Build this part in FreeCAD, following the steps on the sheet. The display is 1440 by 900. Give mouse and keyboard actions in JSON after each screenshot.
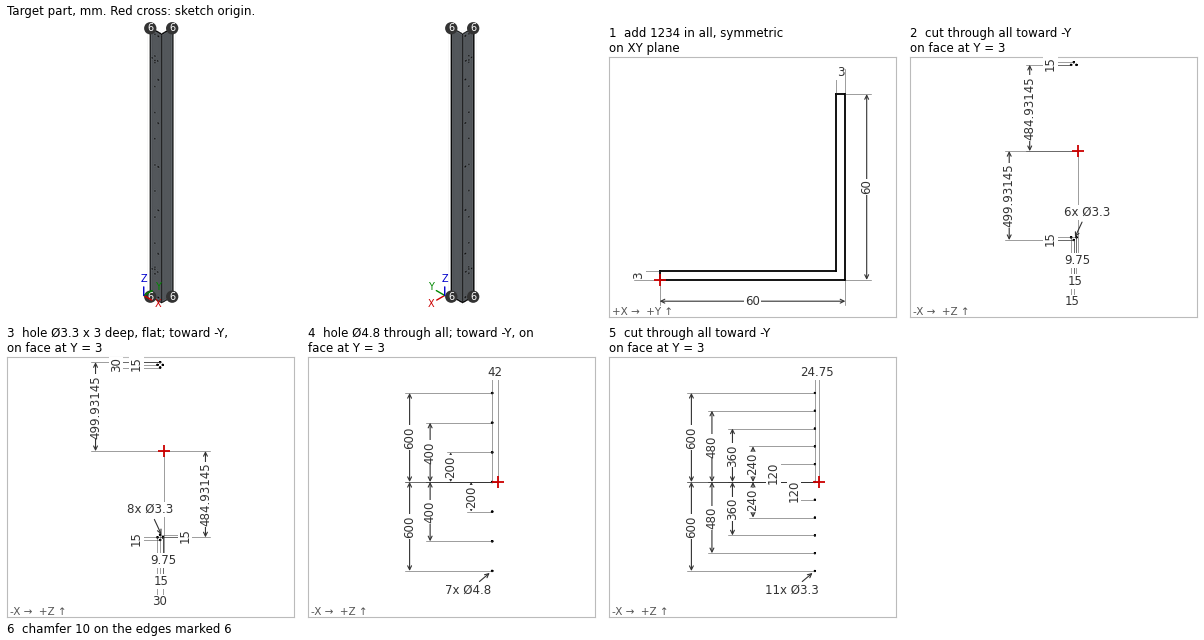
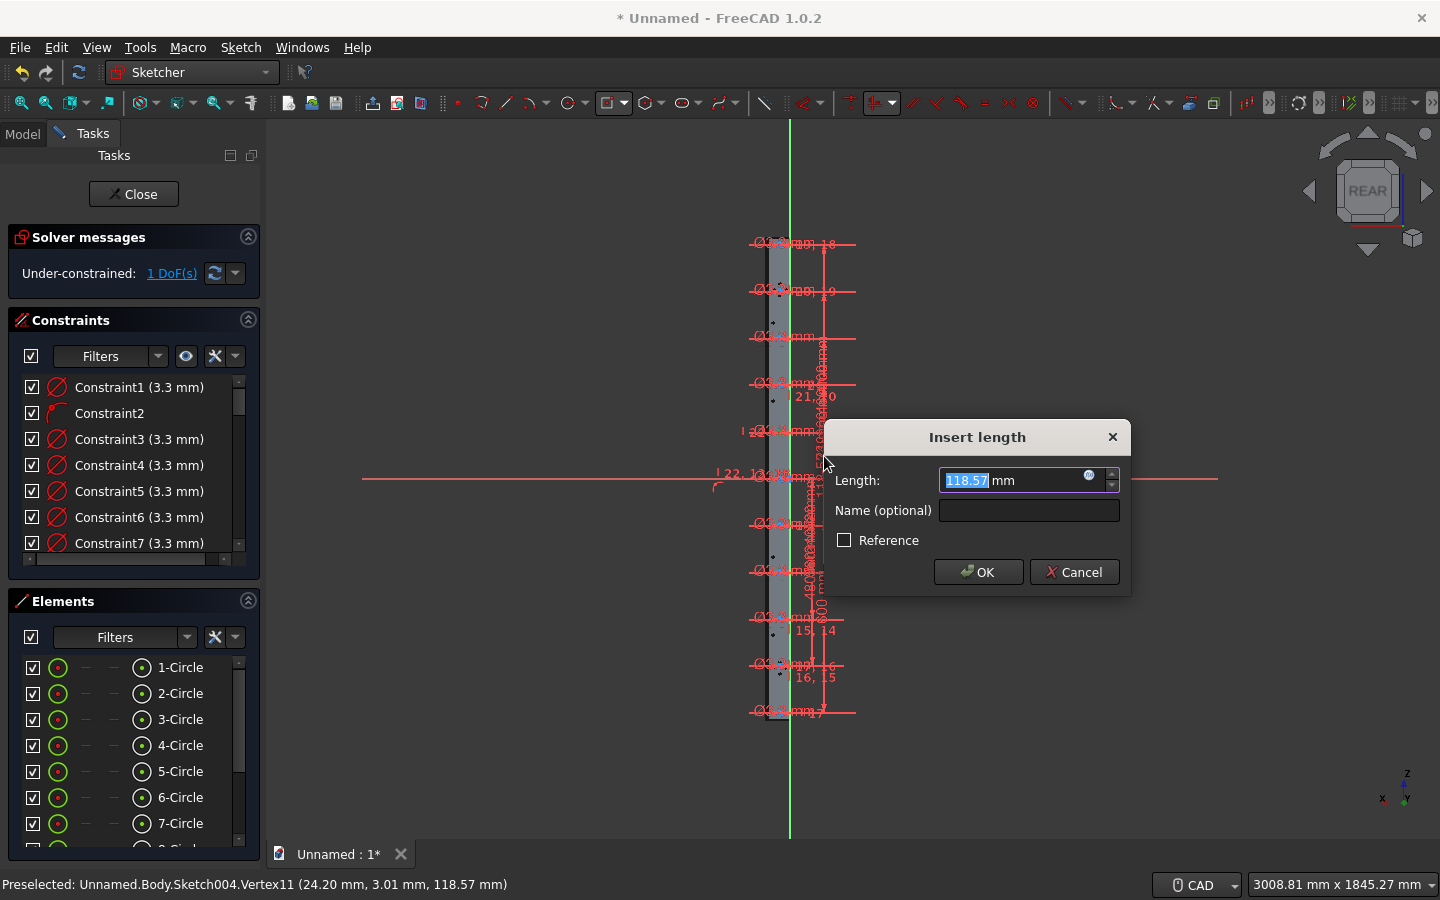
{"action": "type", "text": "120"}
{"action": "key", "text": "Return"}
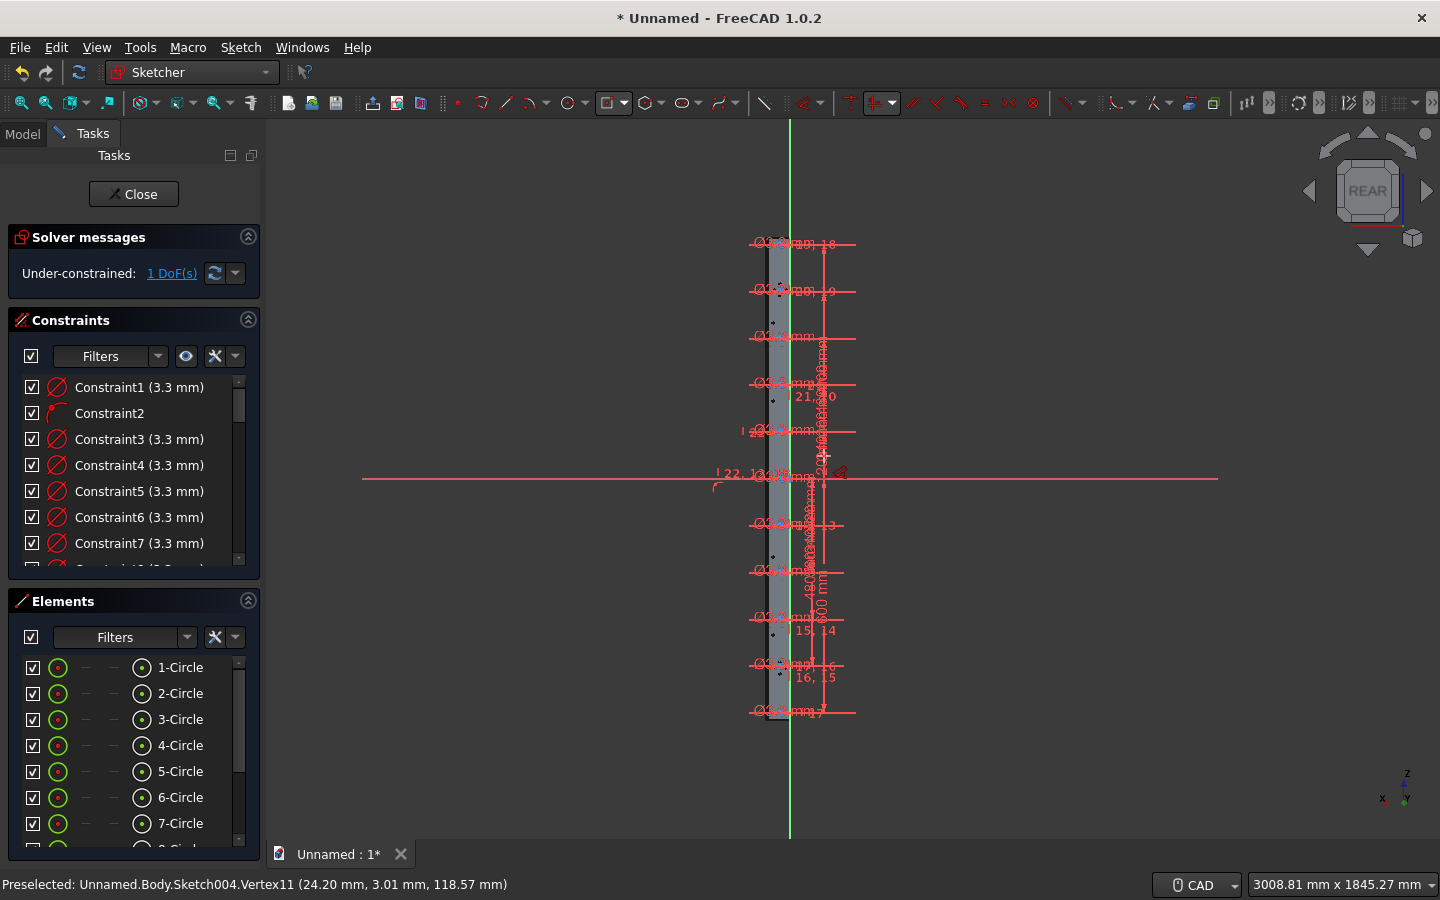
{"action": "scroll", "coordinate": [780, 479], "scroll_direction": "up", "scroll_amount": 8}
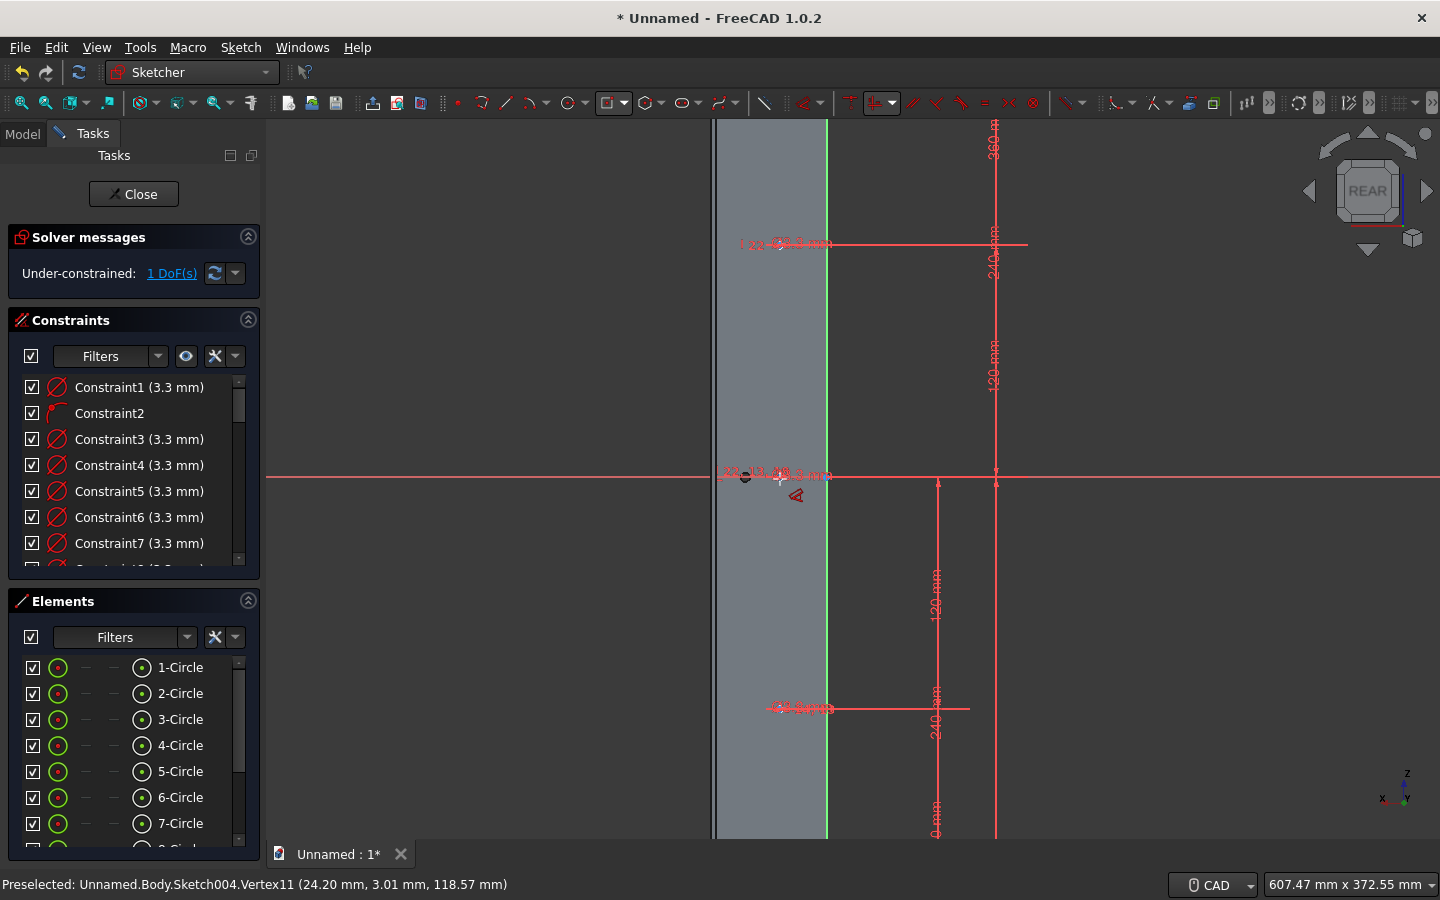
{"action": "left_click", "coordinate": [780, 477]}
{"action": "left_click", "coordinate": [803, 511]}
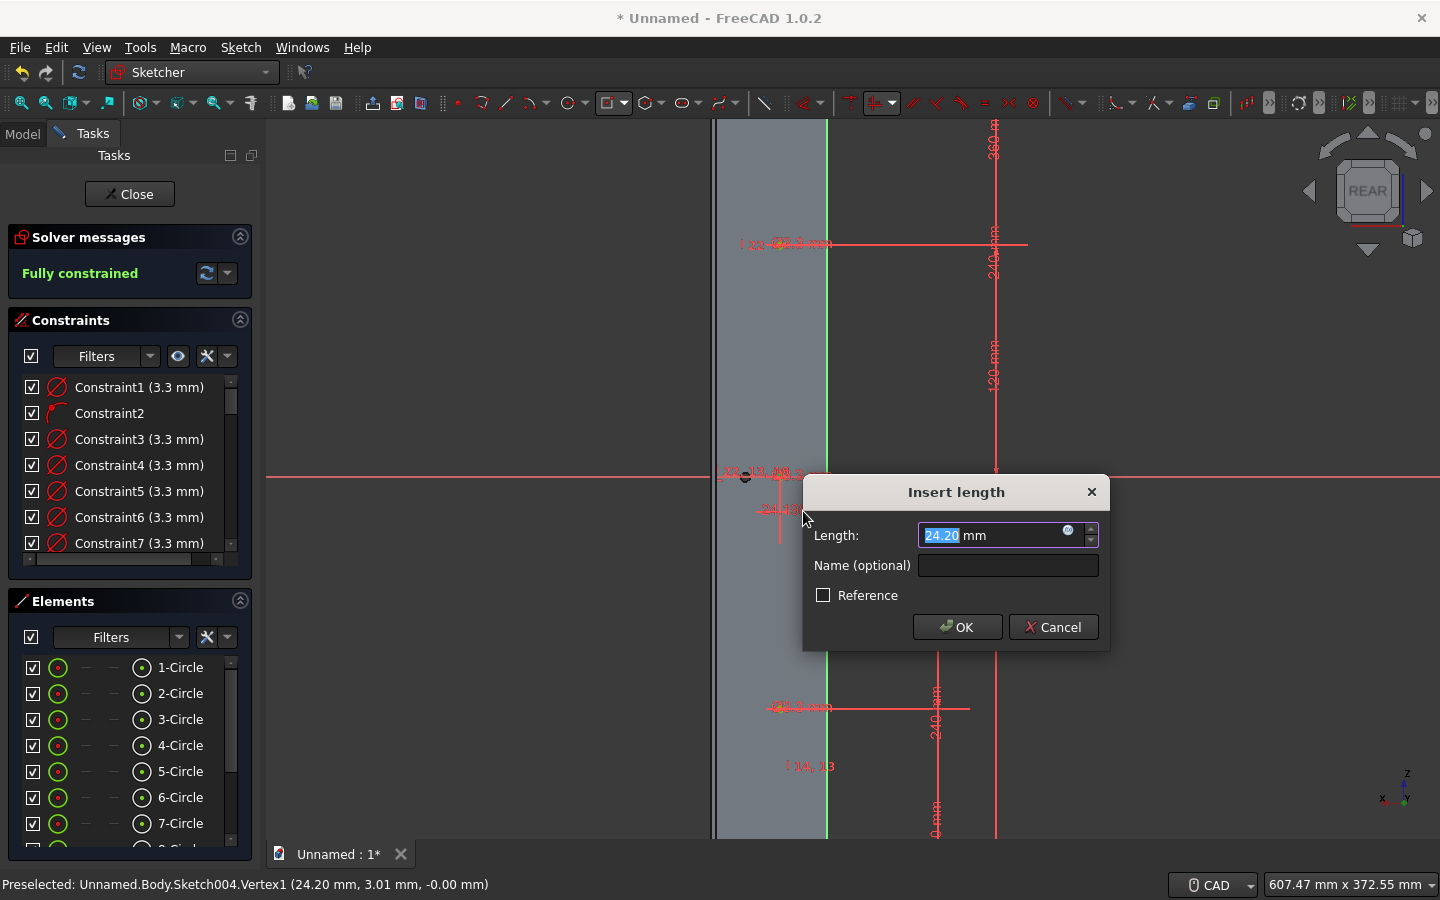
{"action": "type", "text": "24.75"}
{"action": "key", "text": "Return"}
{"action": "key", "text": "Escape"}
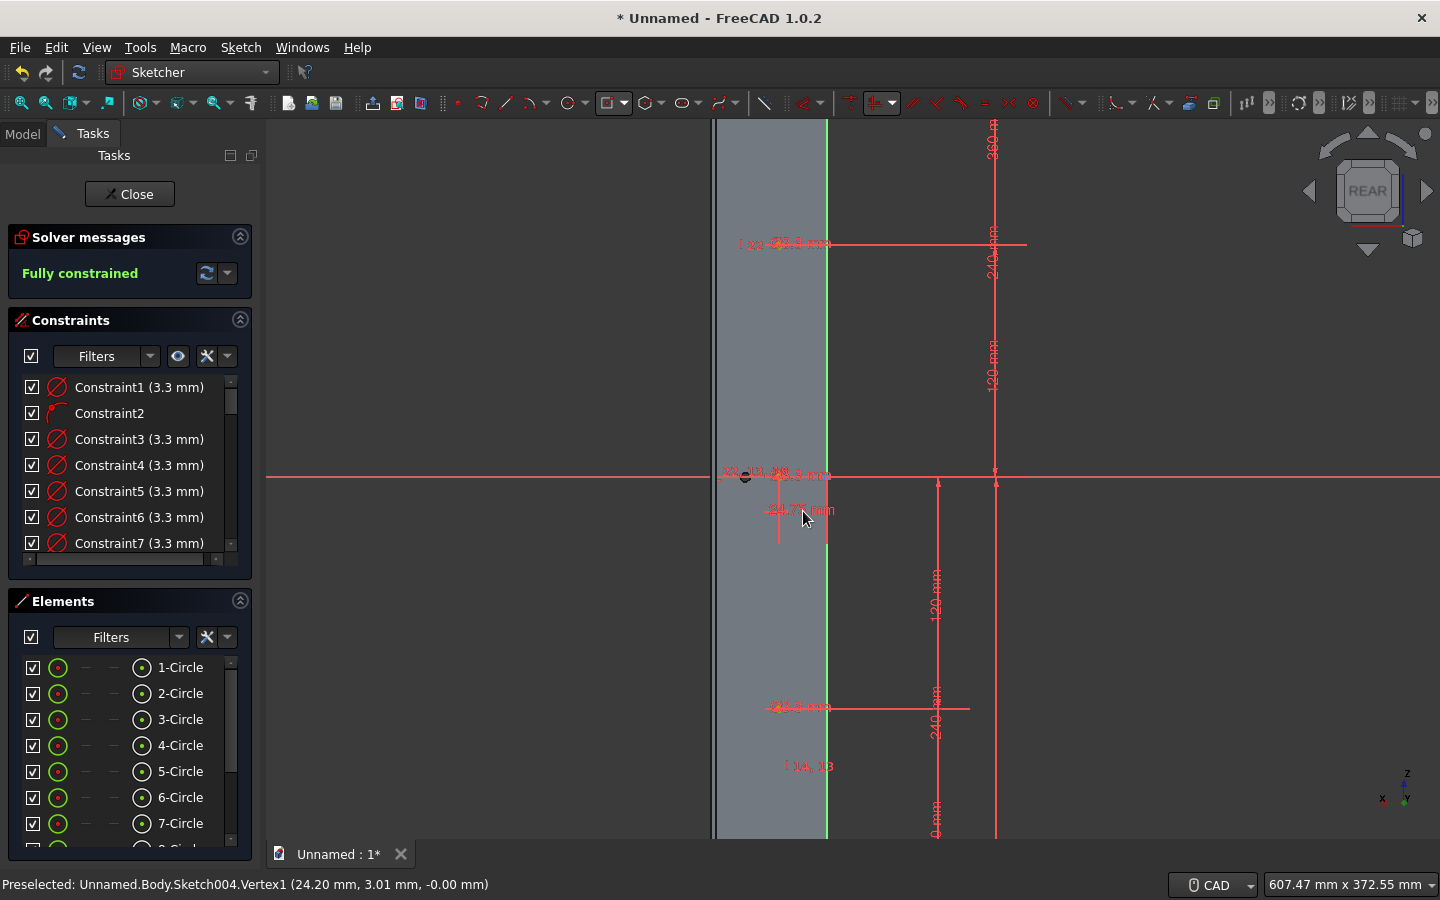
{"action": "left_click", "coordinate": [130, 194]}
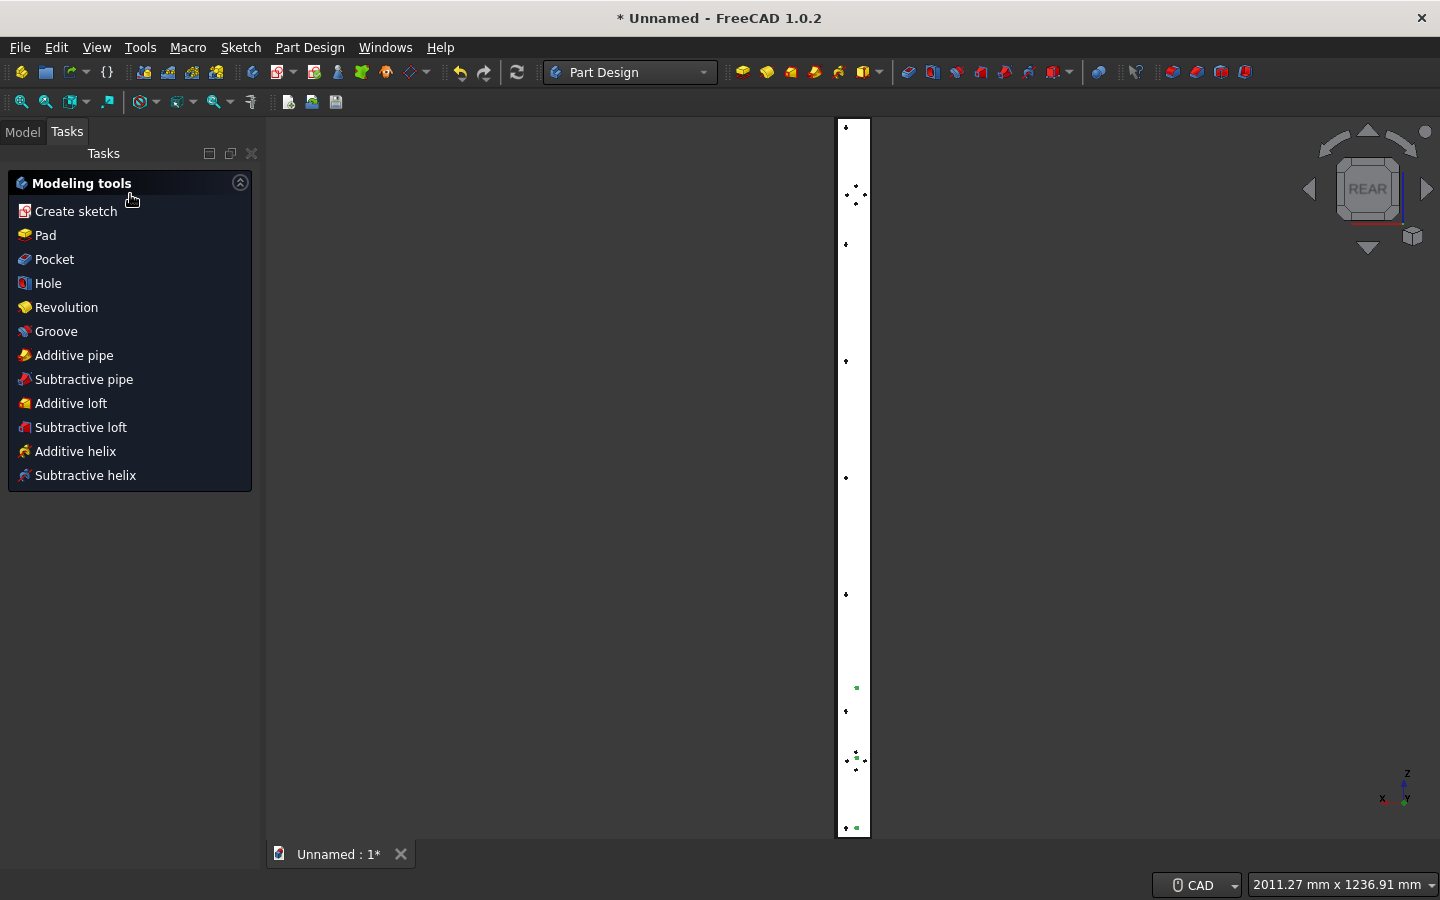
{"action": "left_click", "coordinate": [910, 72]}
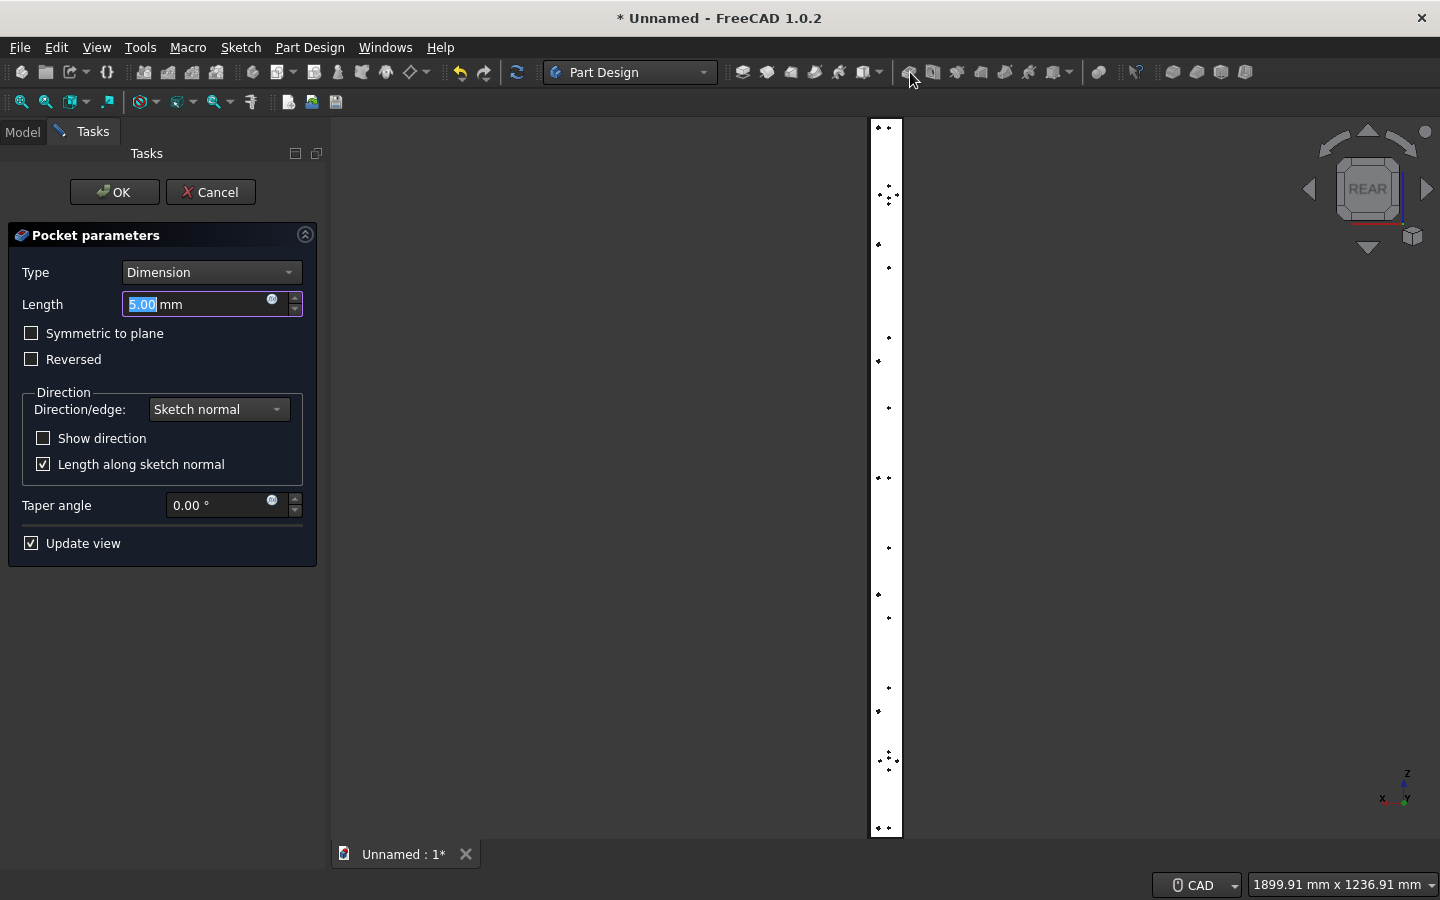
{"action": "left_click", "coordinate": [212, 272]}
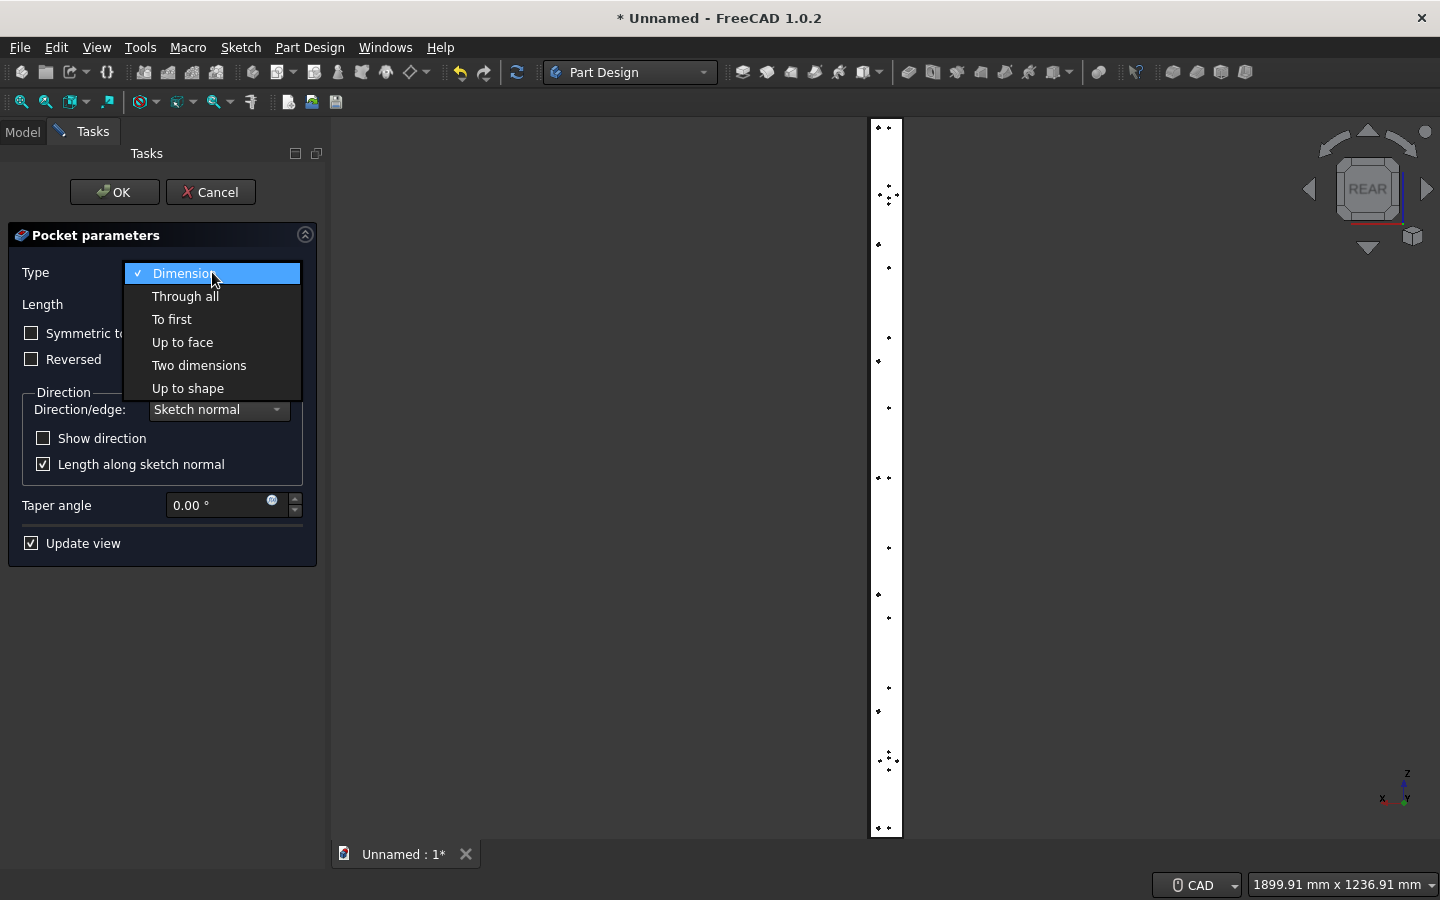
{"action": "left_click", "coordinate": [212, 296]}